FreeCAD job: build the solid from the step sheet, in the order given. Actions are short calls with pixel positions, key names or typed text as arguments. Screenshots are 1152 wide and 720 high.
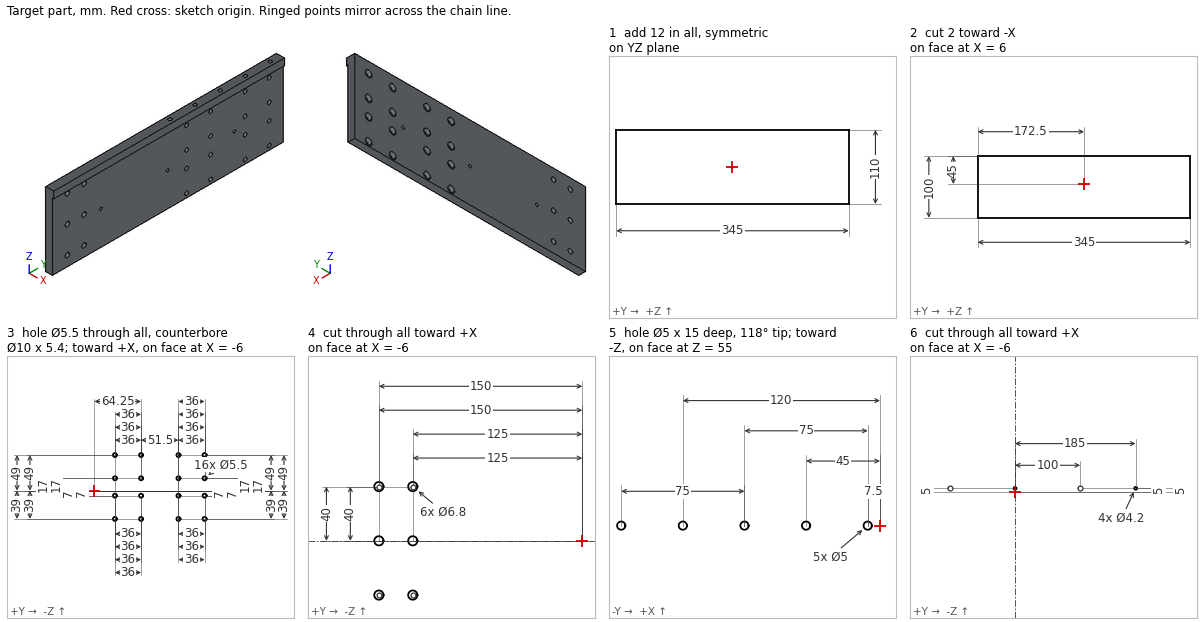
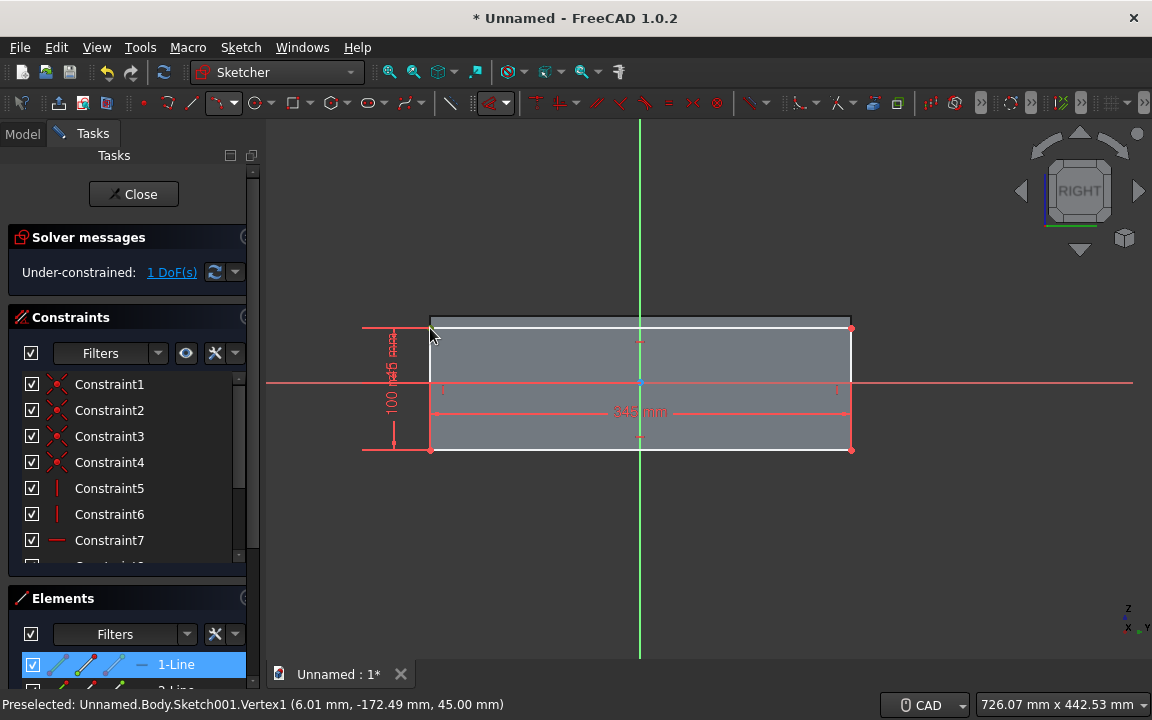
key(l)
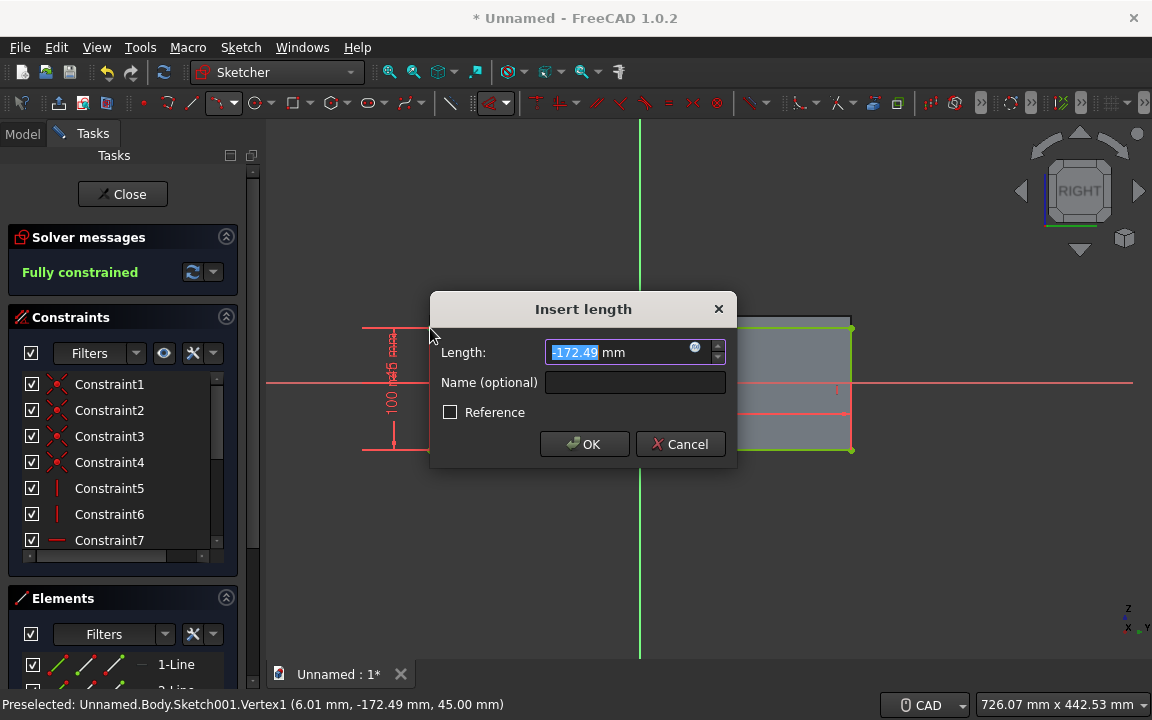
text(-172.5)
key(Return)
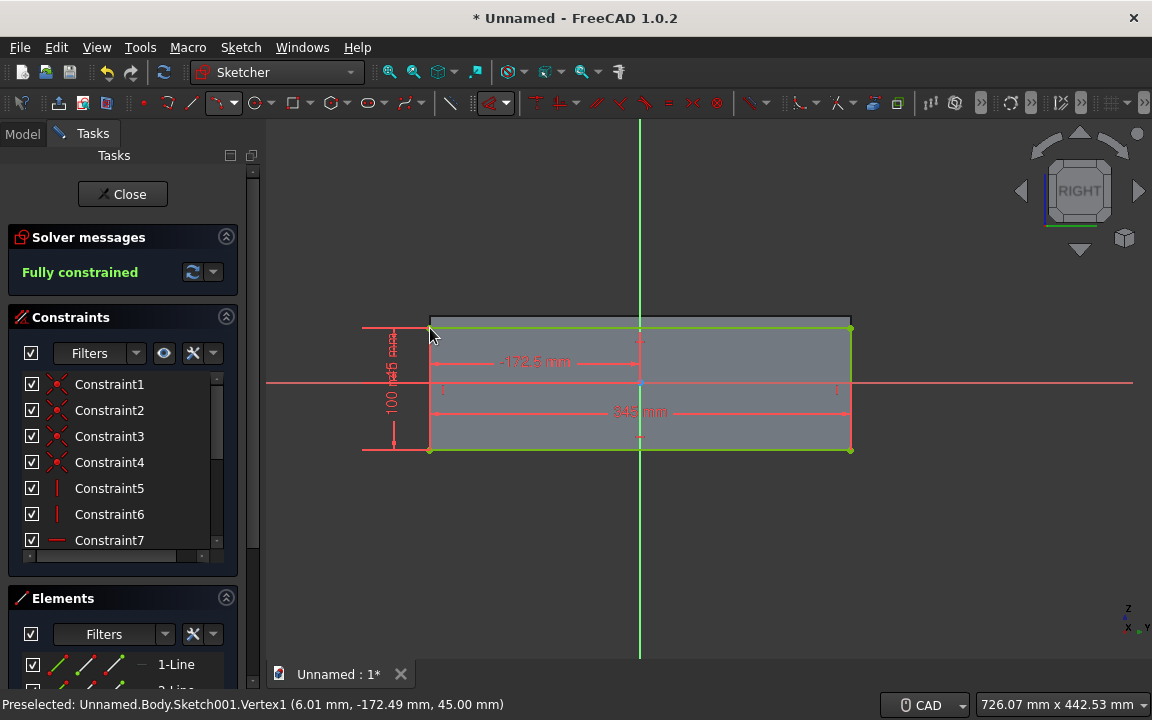
click(123, 194)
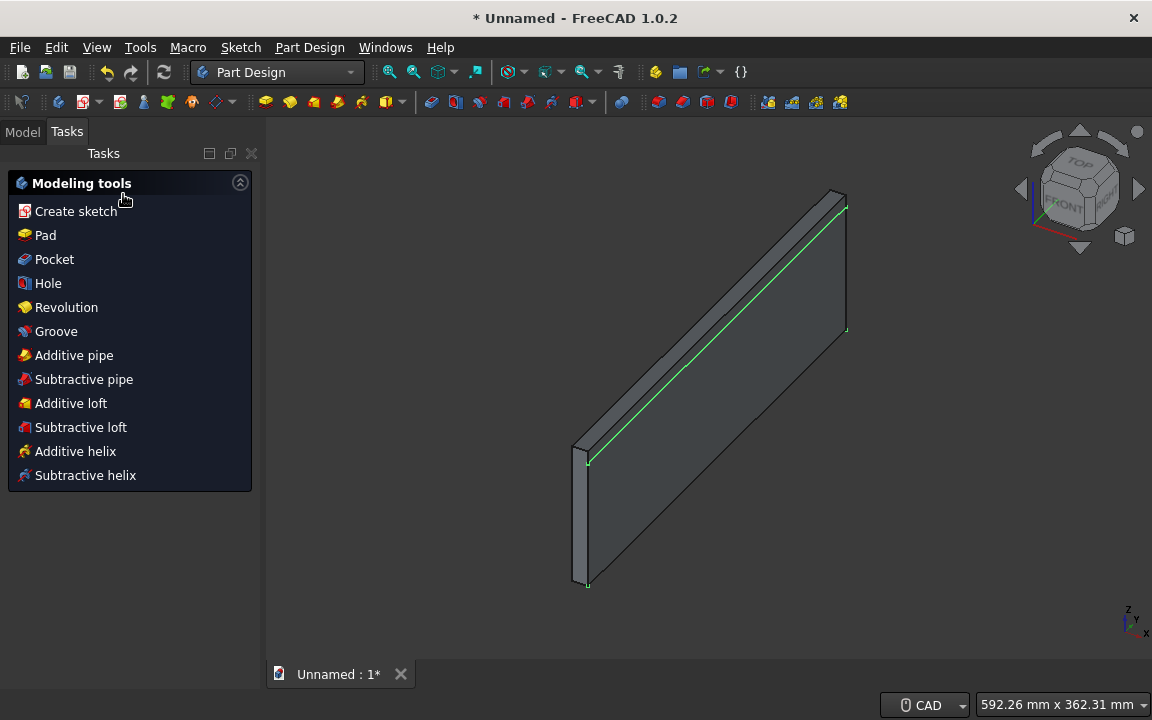
click(432, 102)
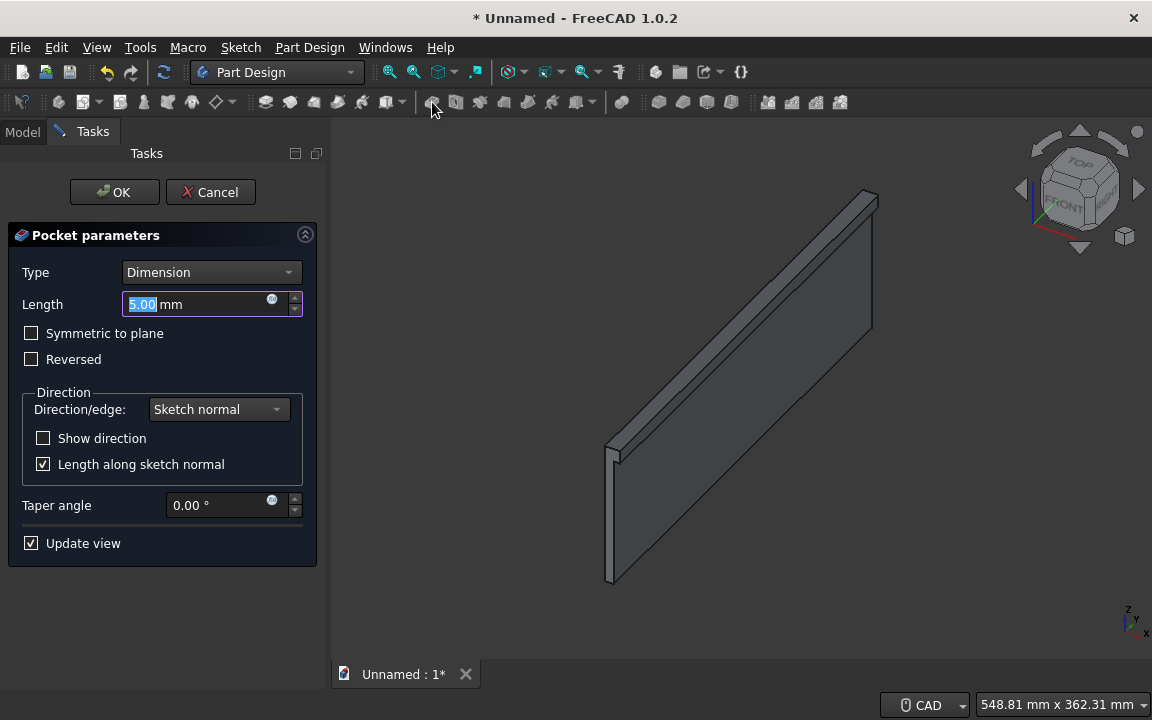
text(2)
key(Tab)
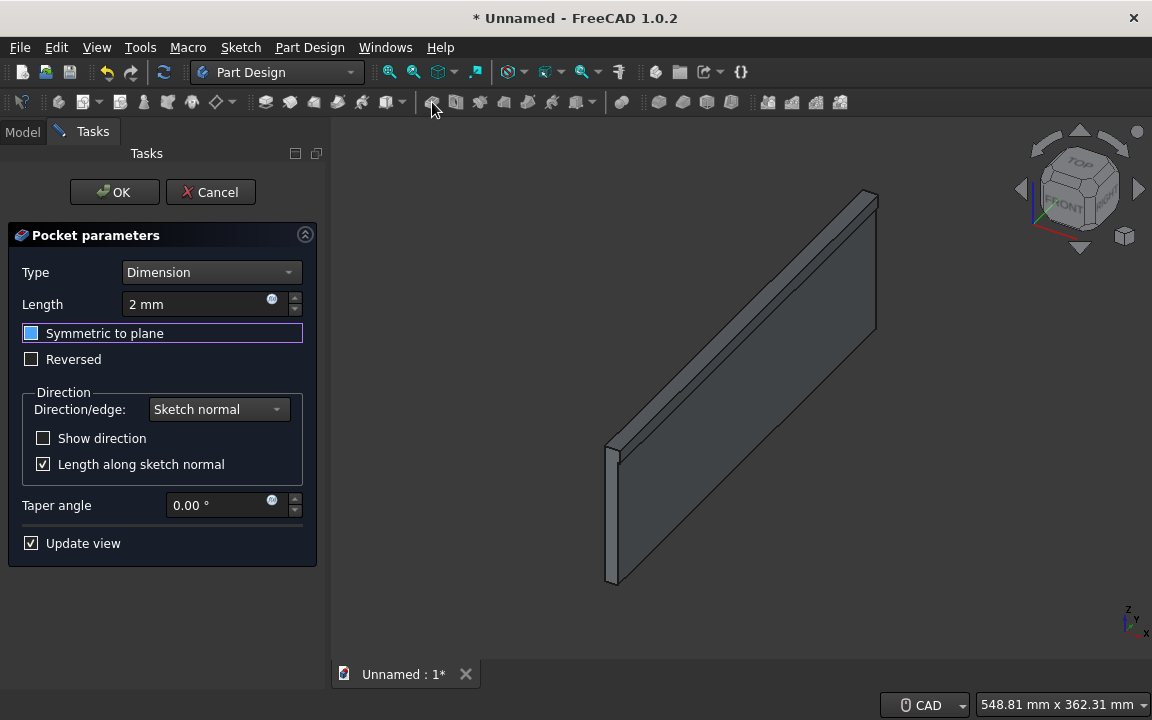
click(115, 192)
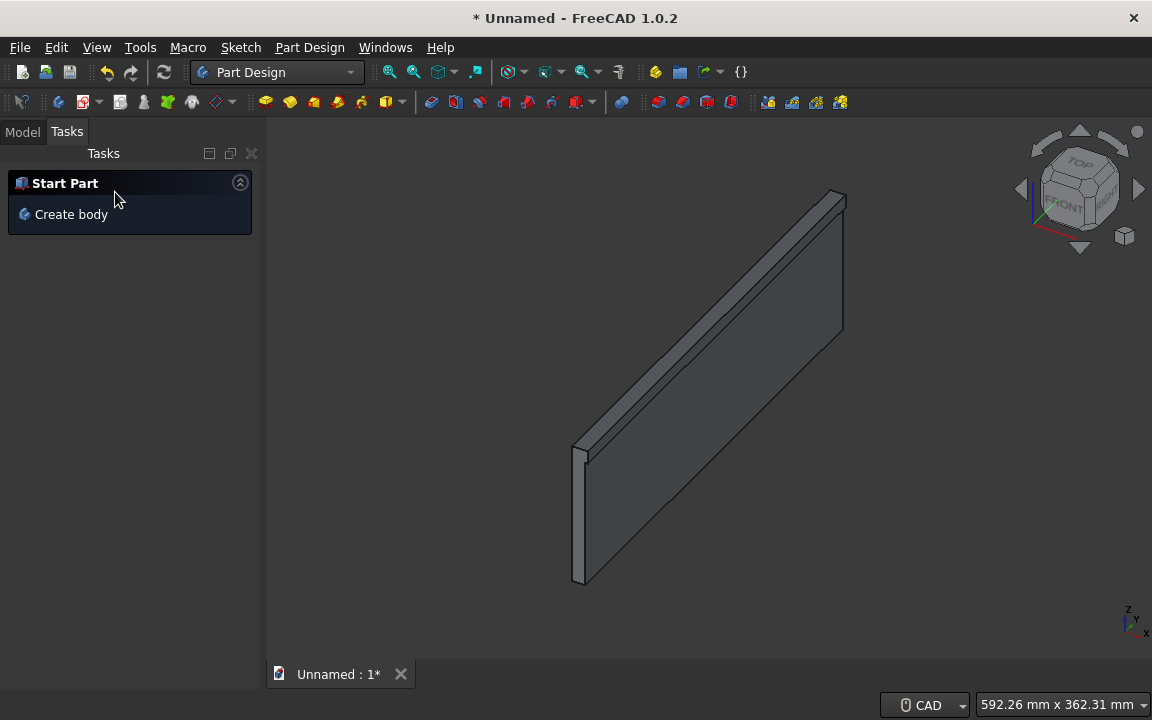
key(6)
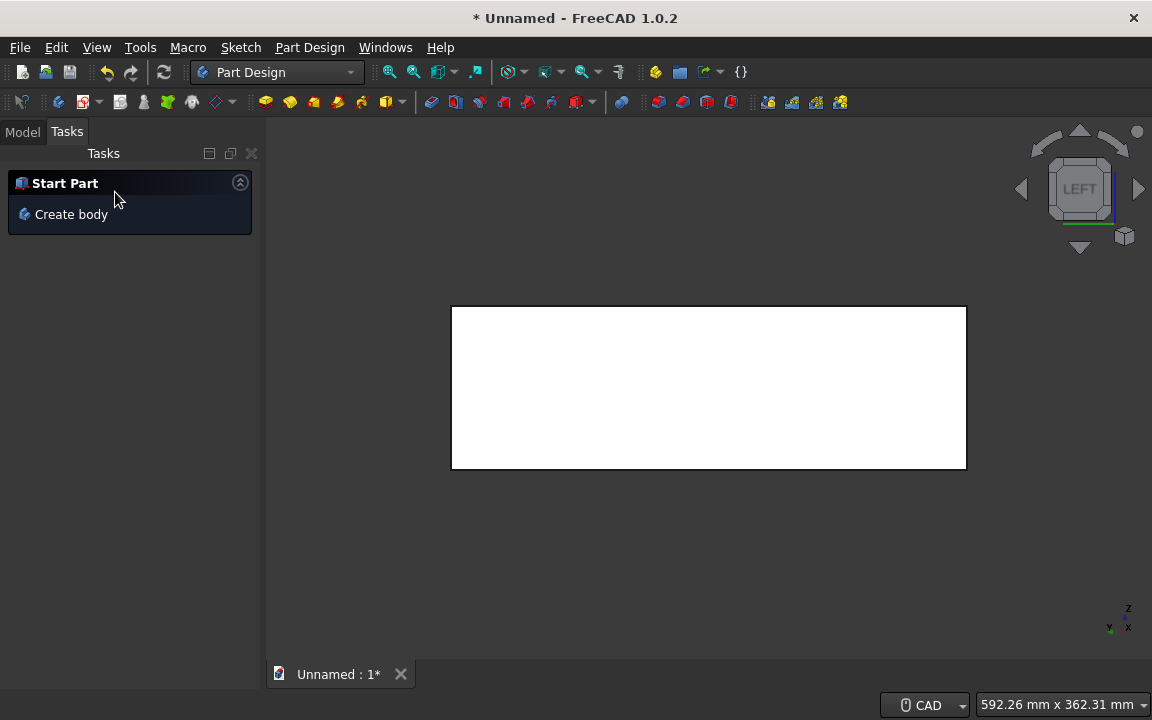
click(562, 387)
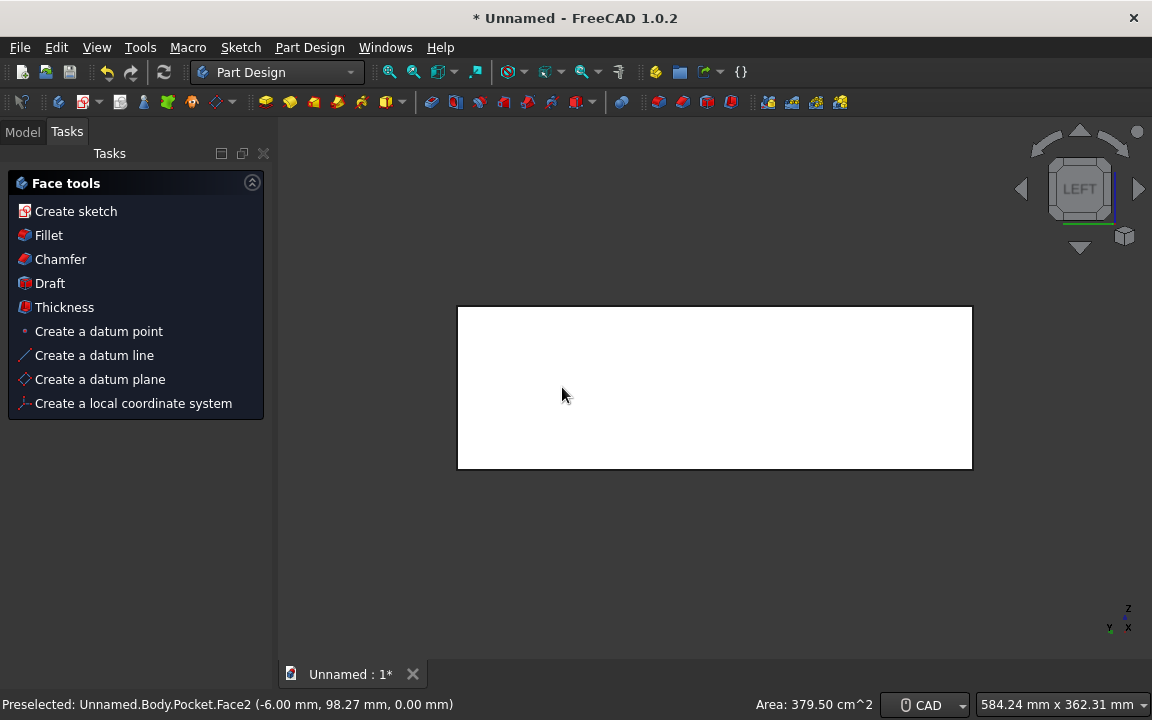
click(84, 102)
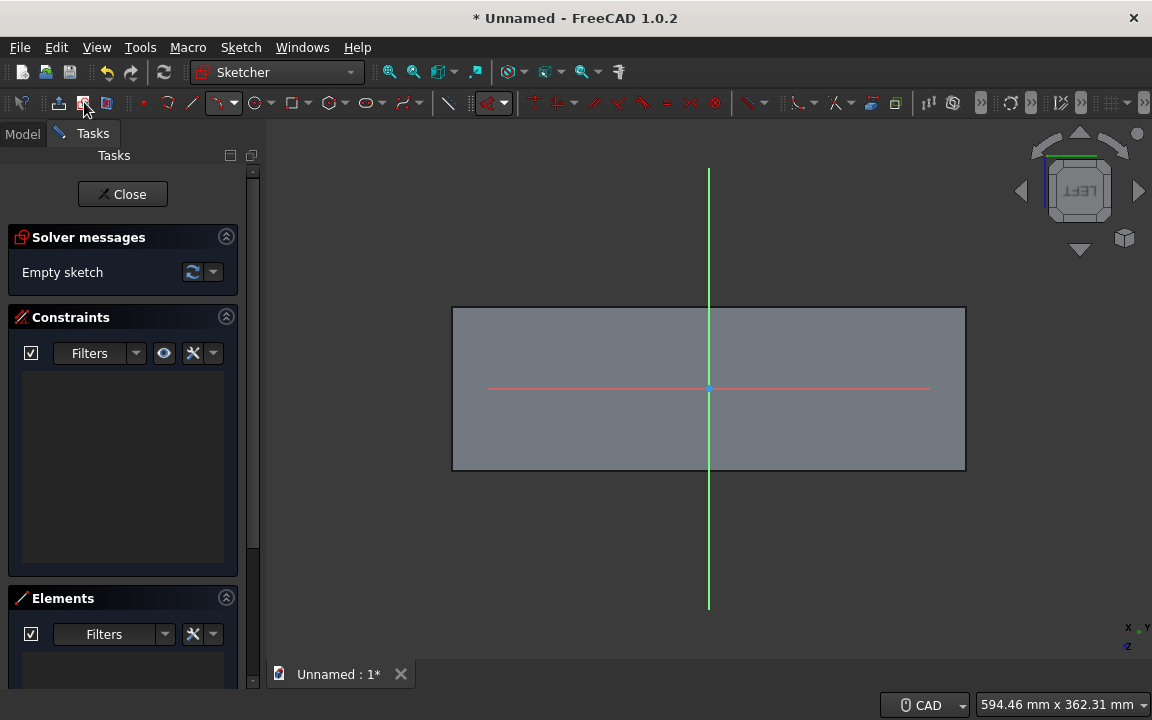
scroll(974, 375, up, 4)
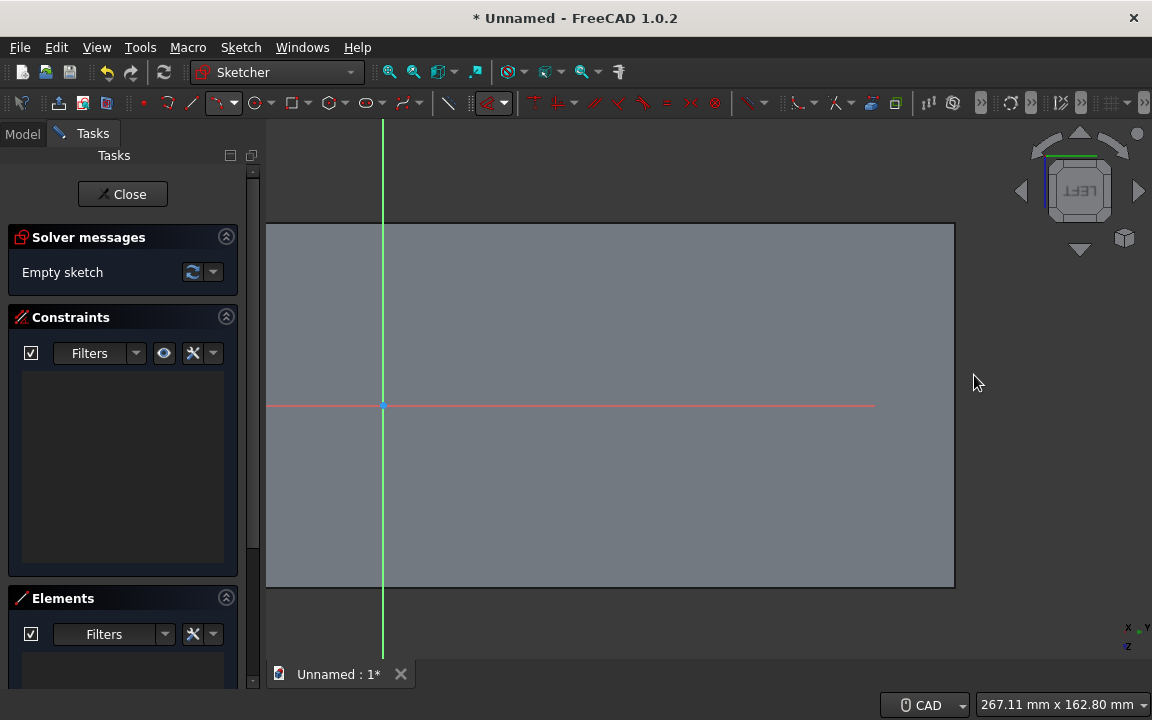
click(256, 104)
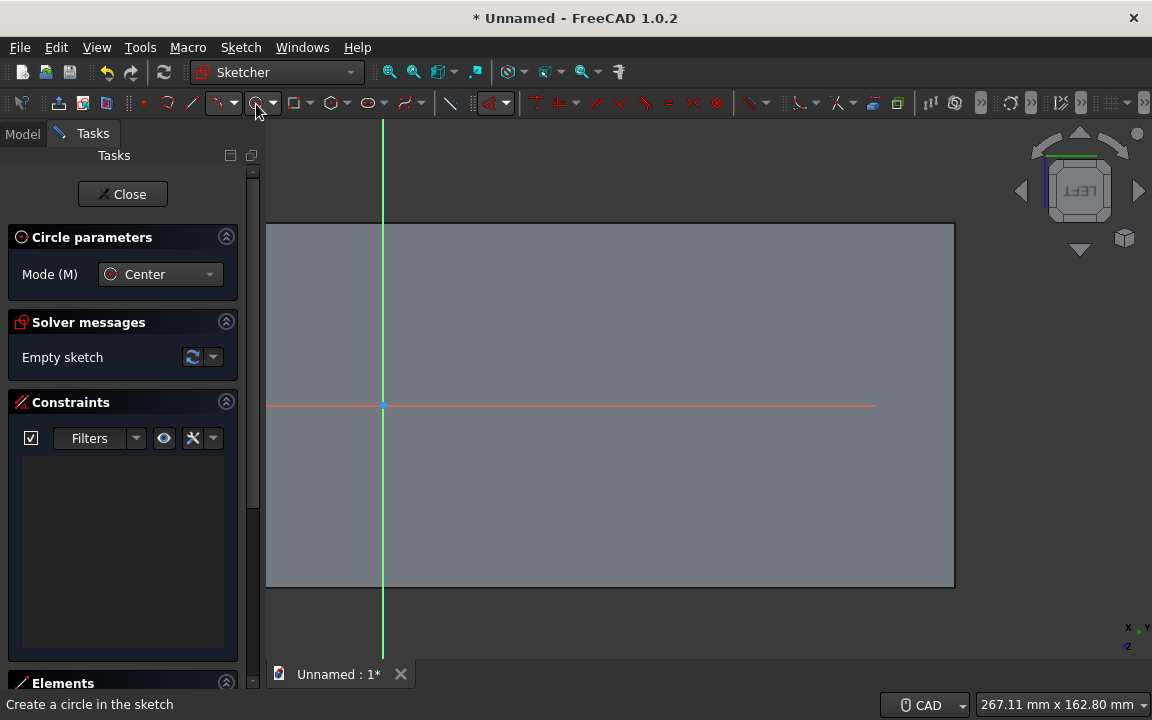
scroll(887, 243, up, 5)